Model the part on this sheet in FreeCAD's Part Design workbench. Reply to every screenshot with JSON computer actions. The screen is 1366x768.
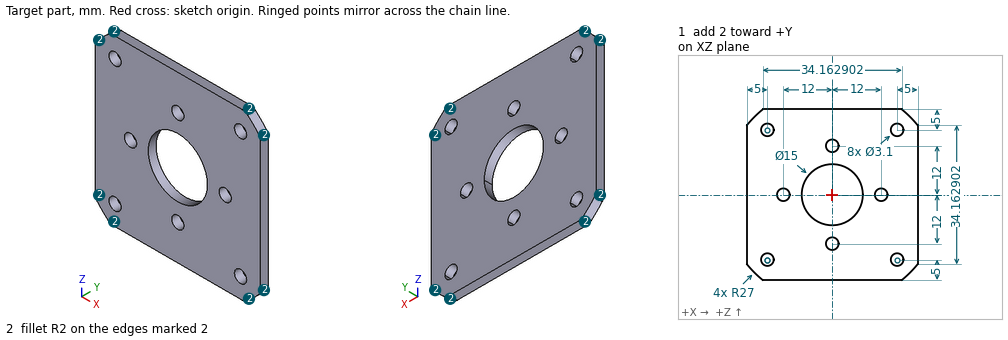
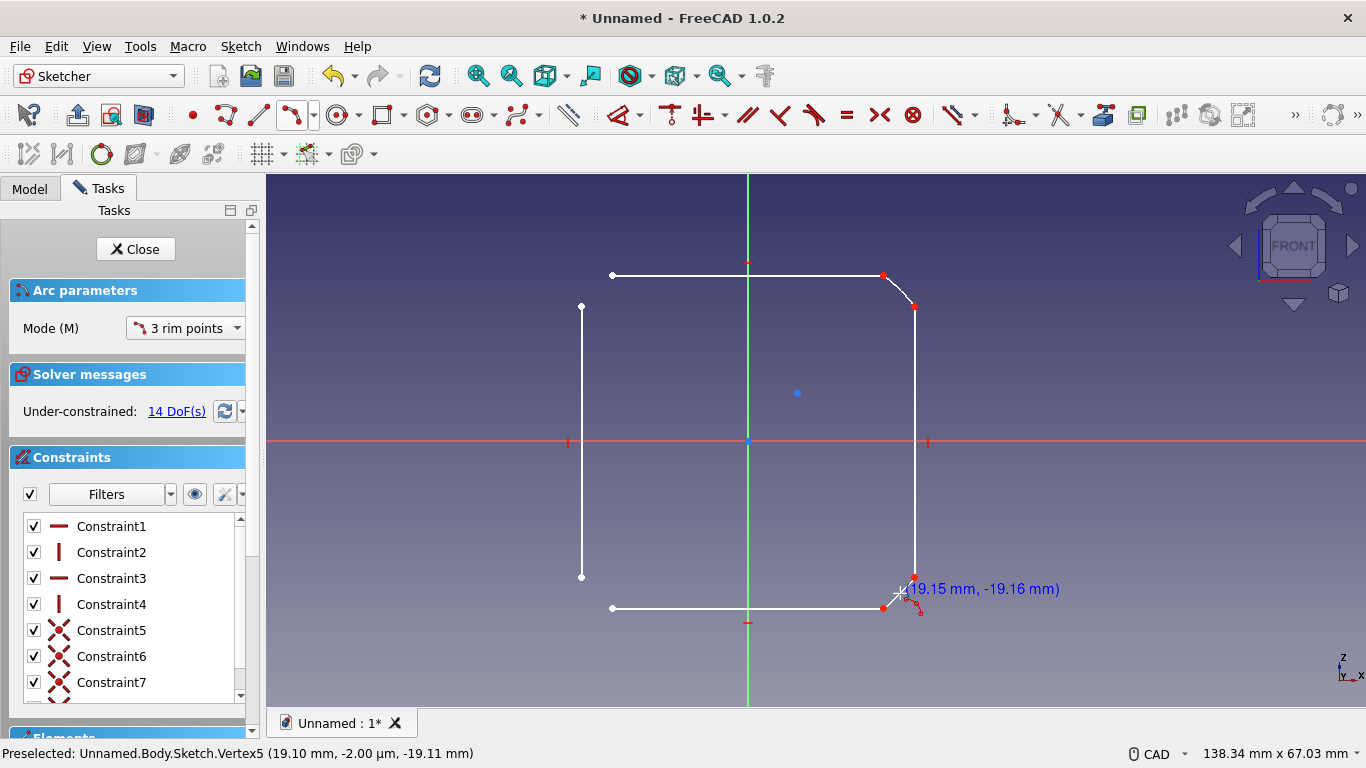
{"action": "left_click", "coordinate": [613, 609]}
{"action": "left_click", "coordinate": [582, 578]}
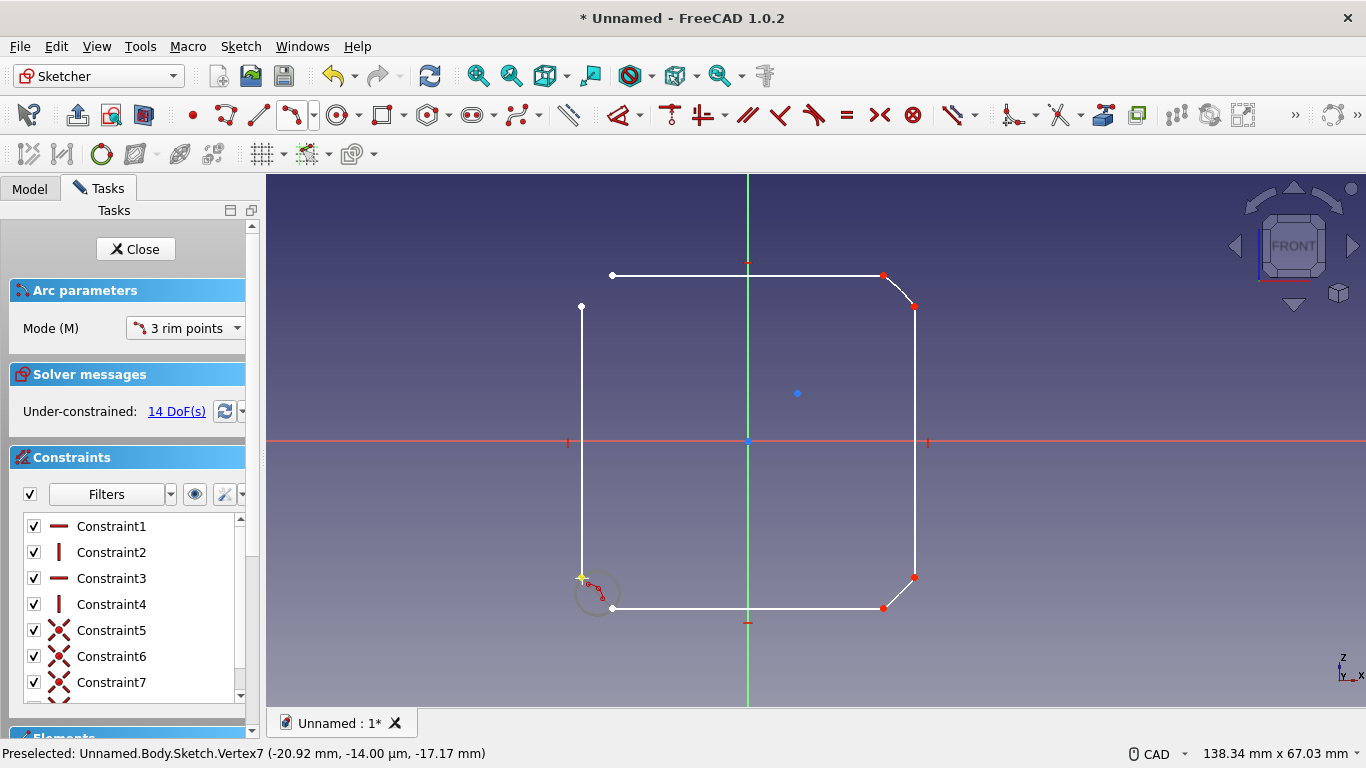
{"action": "scroll", "coordinate": [596, 593], "scroll_direction": "up", "scroll_amount": 14}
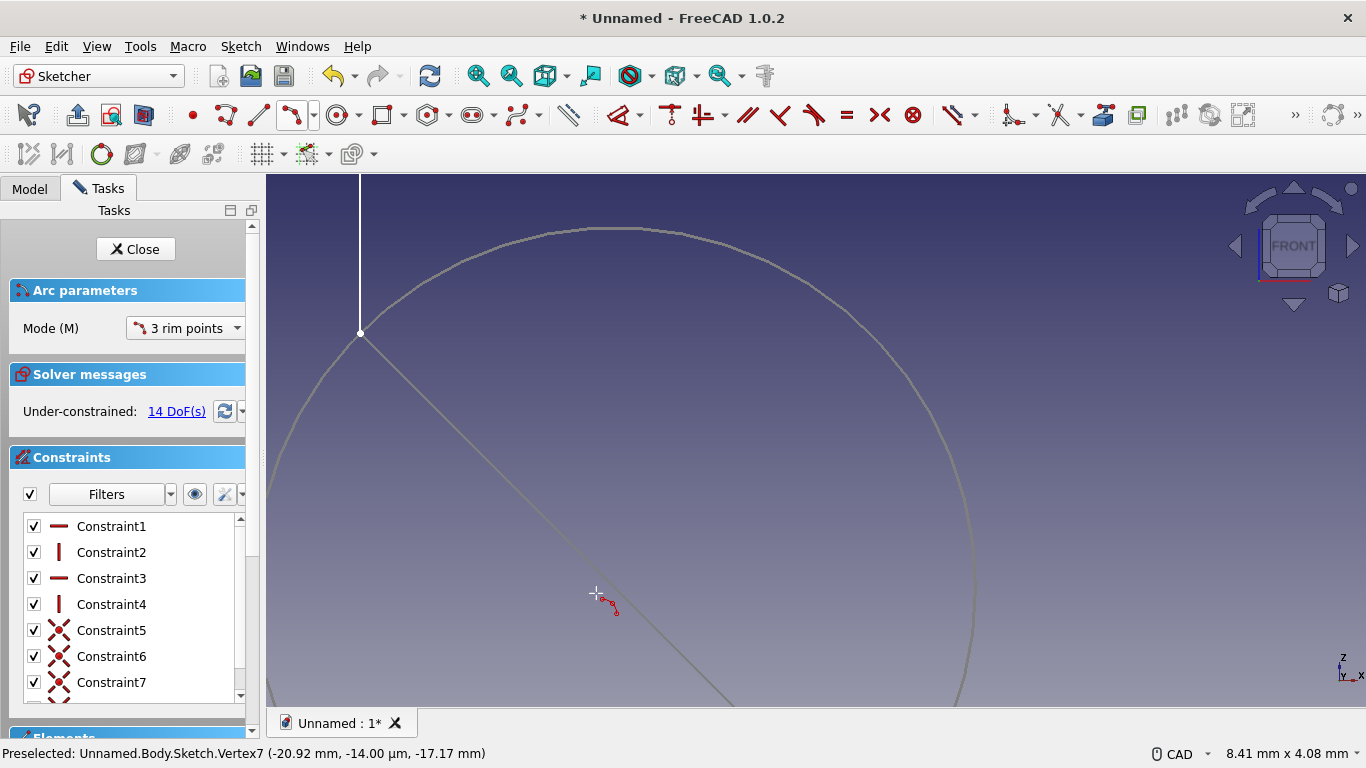
{"action": "left_click", "coordinate": [599, 585]}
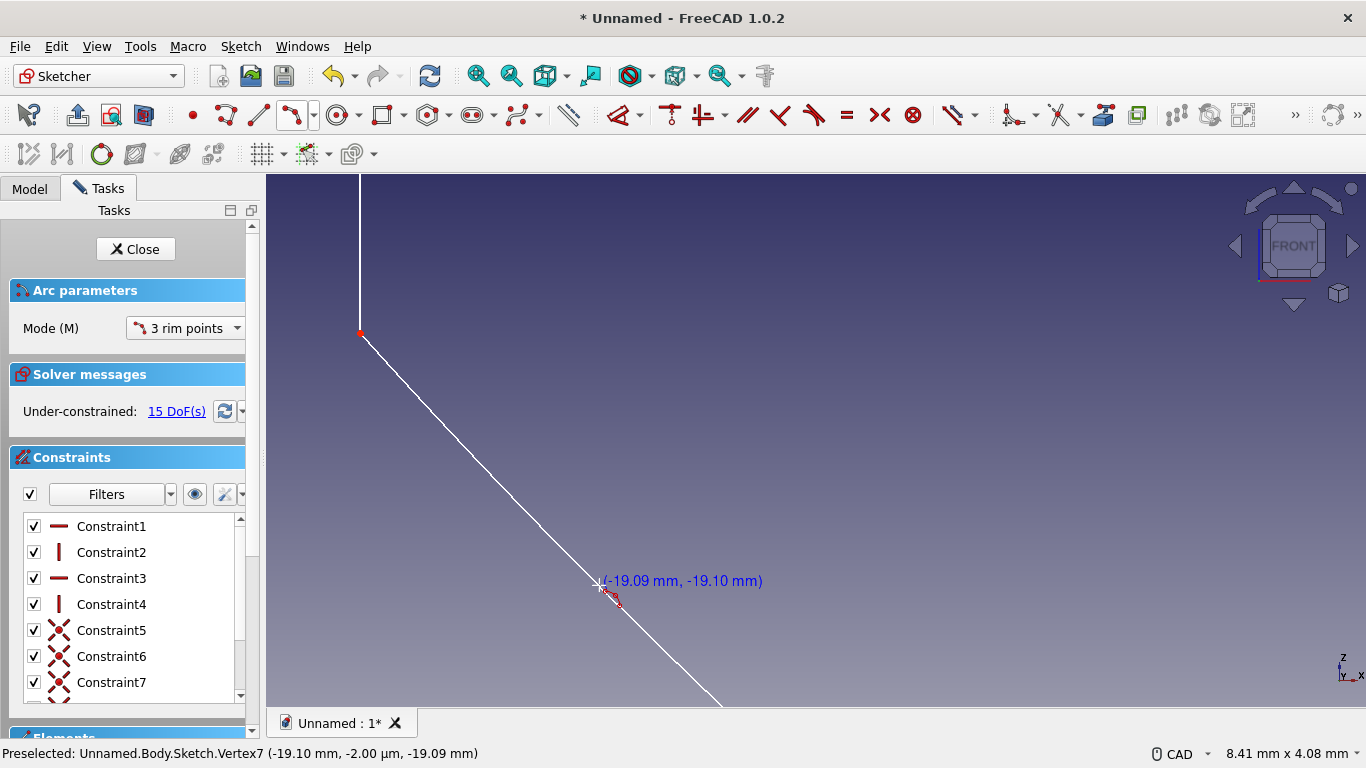
{"action": "scroll", "coordinate": [595, 593], "scroll_direction": "down", "scroll_amount": 14}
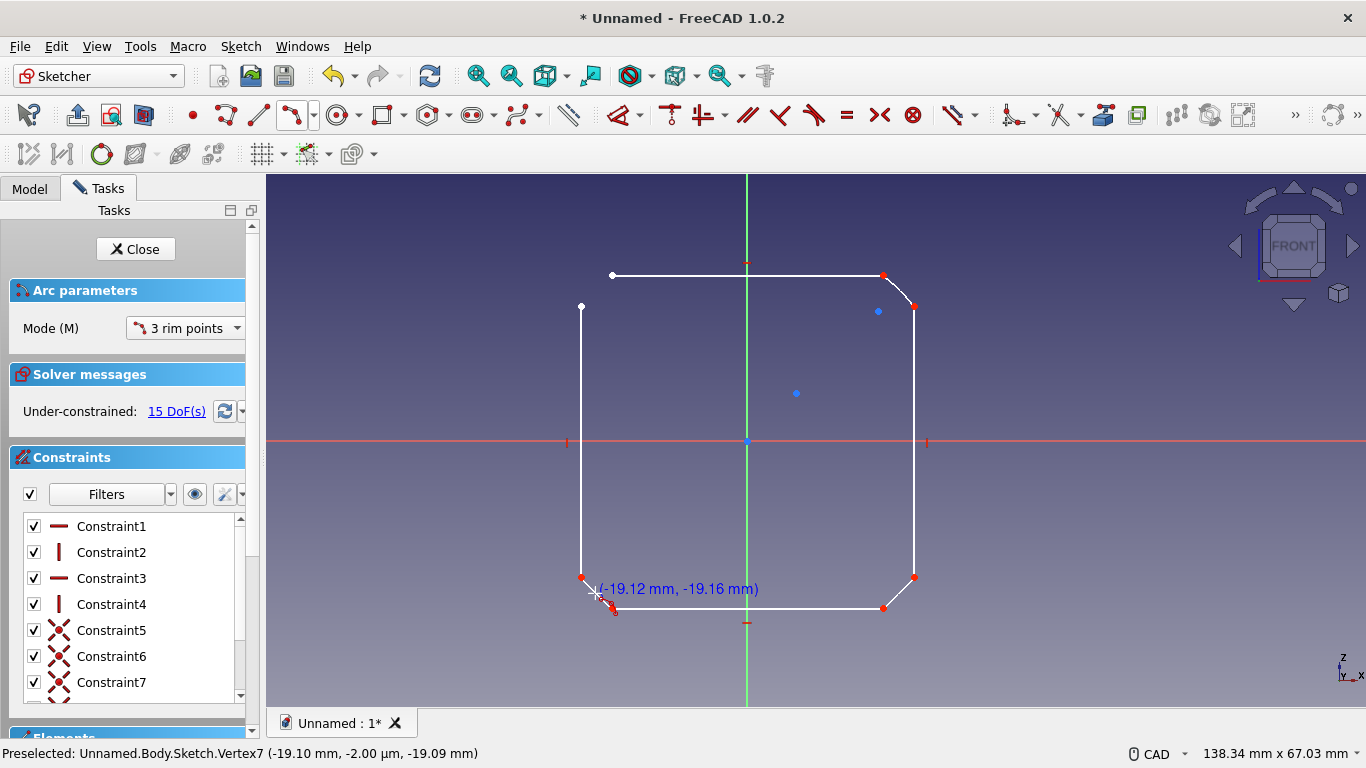
{"action": "left_click", "coordinate": [581, 307]}
{"action": "left_click", "coordinate": [612, 276]}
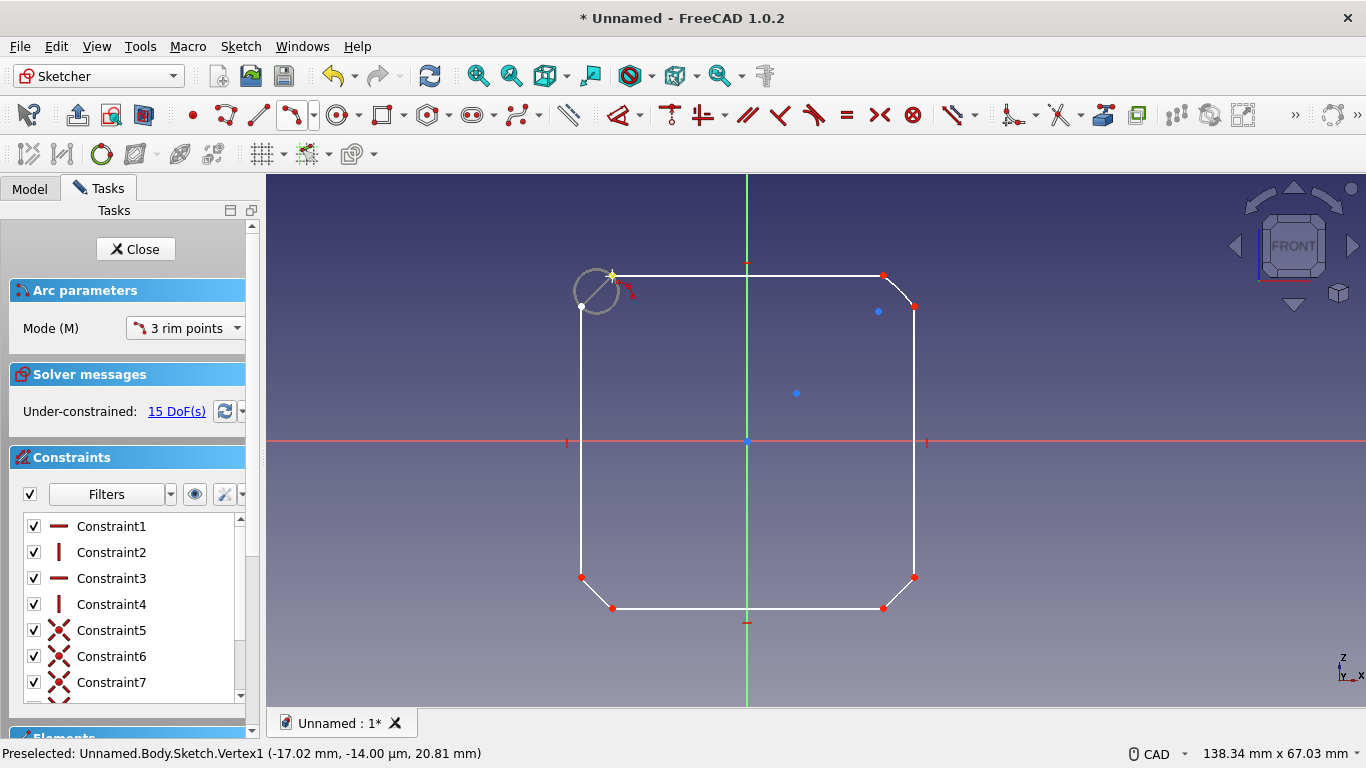
{"action": "scroll", "coordinate": [596, 290], "scroll_direction": "up", "scroll_amount": 14}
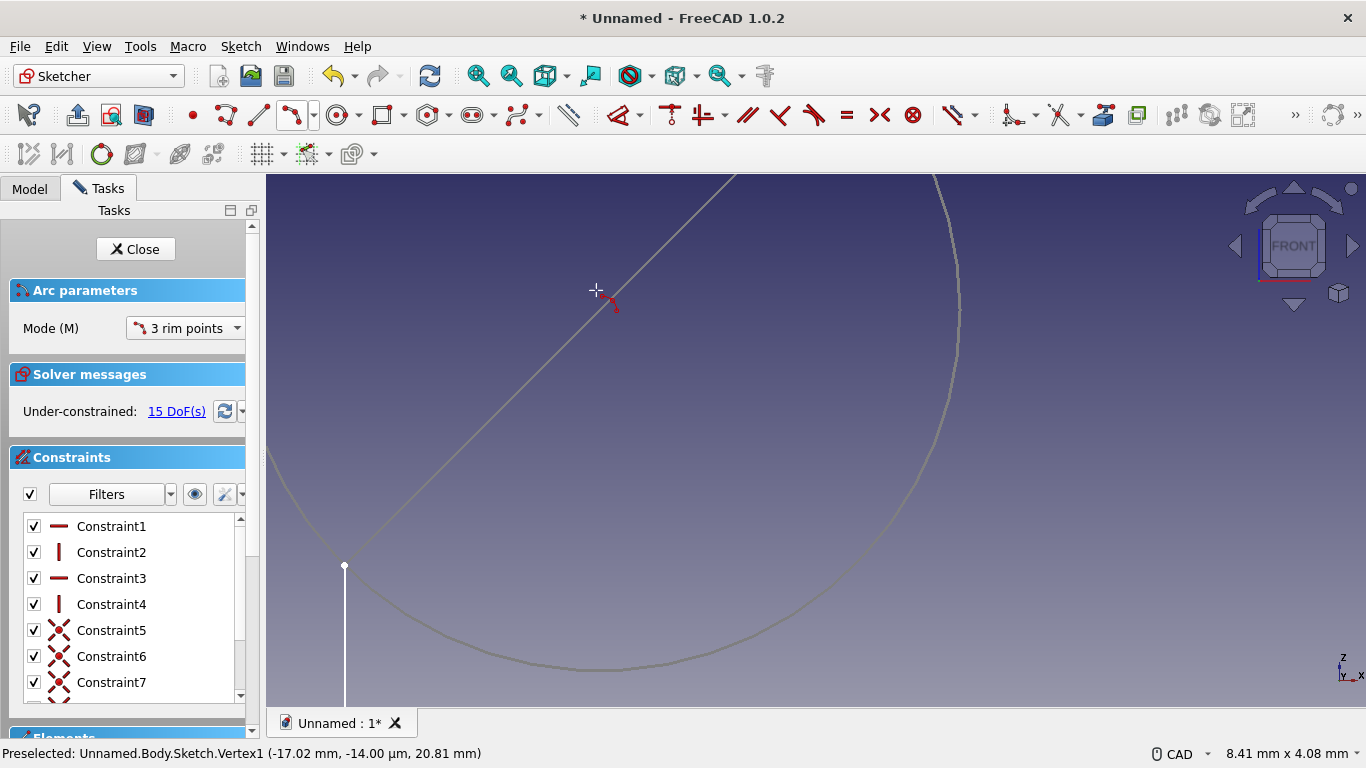
{"action": "left_click", "coordinate": [583, 281]}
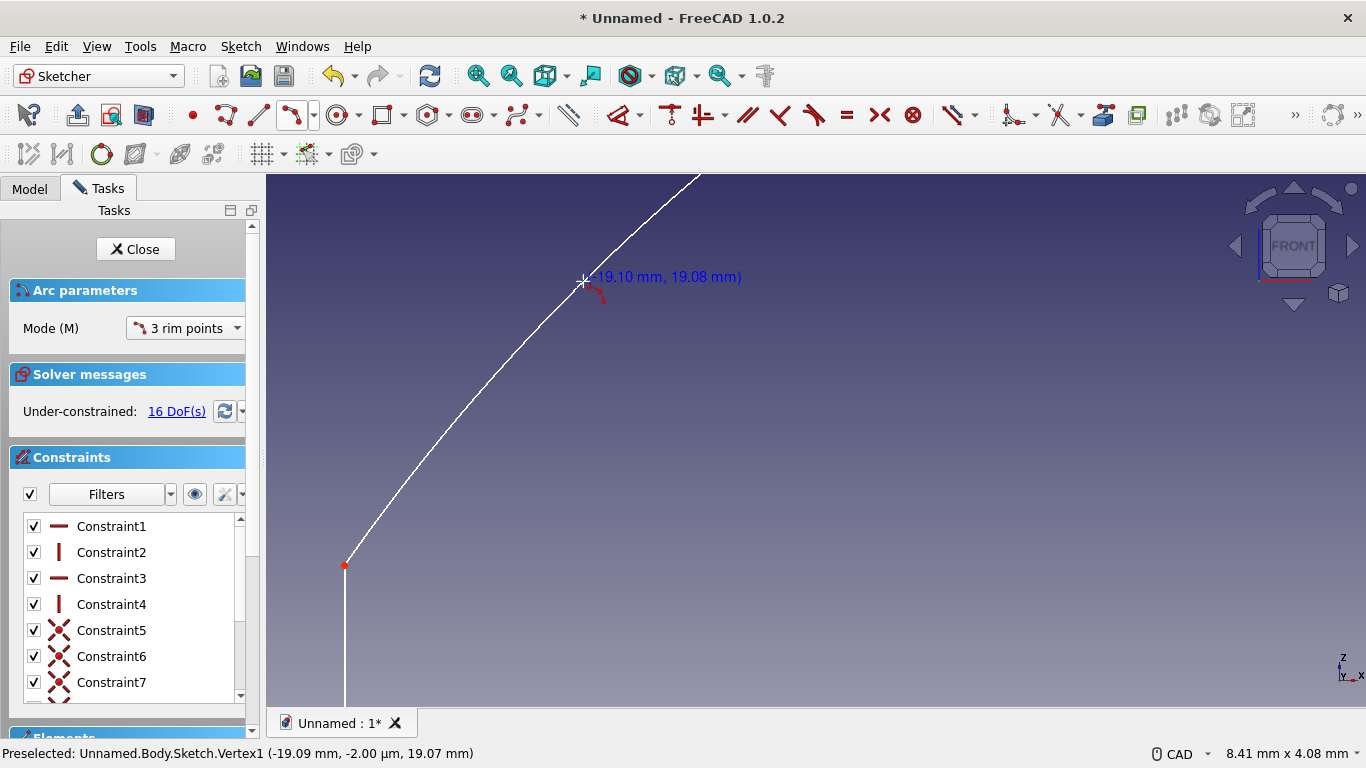
{"action": "left_click", "coordinate": [336, 116]}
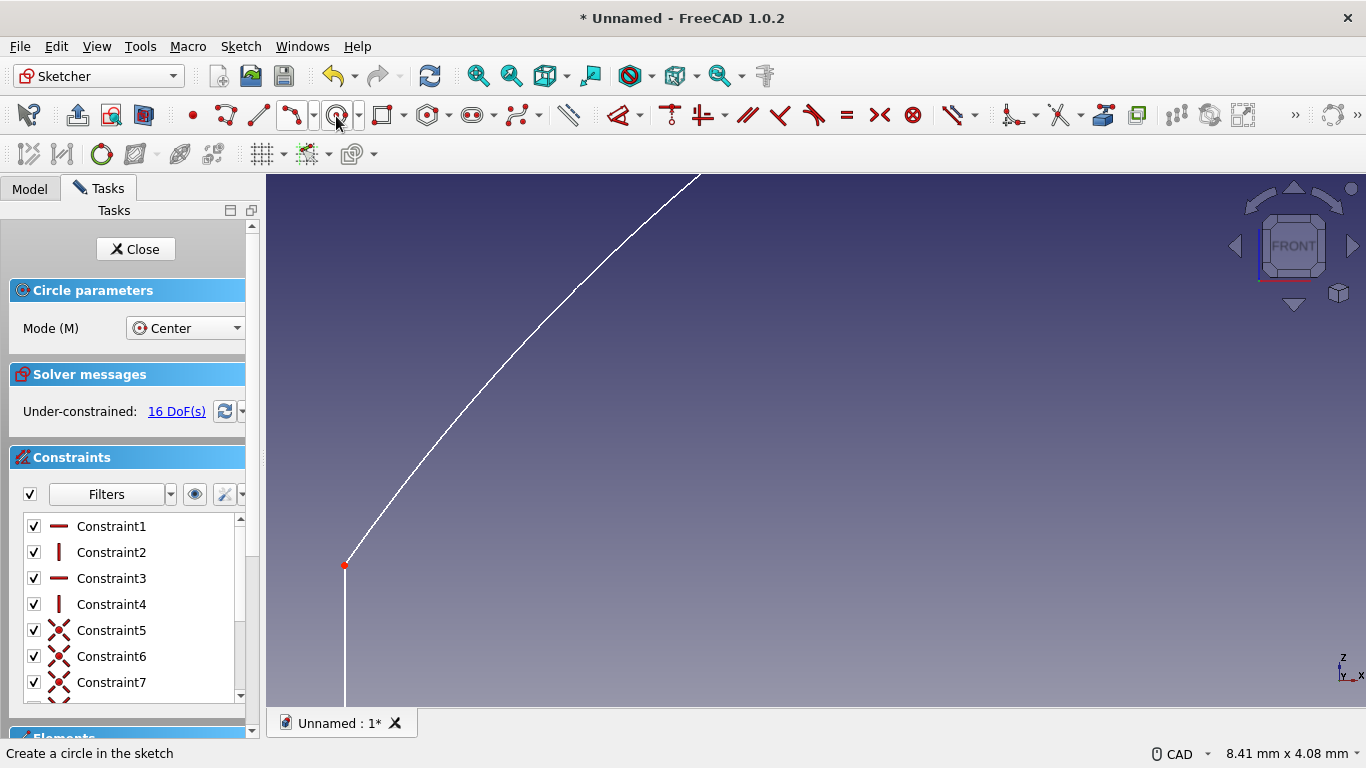
{"action": "scroll", "coordinate": [596, 289], "scroll_direction": "down", "scroll_amount": 14}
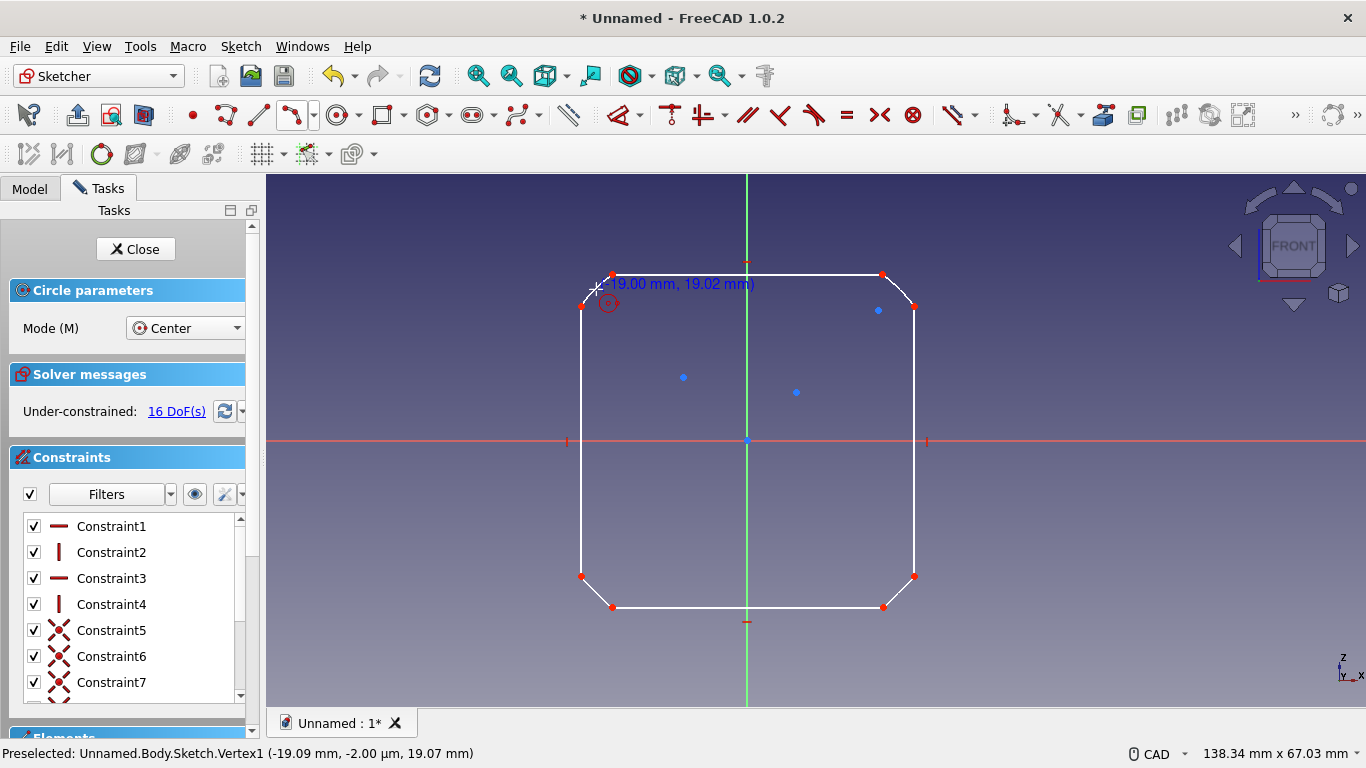
{"action": "scroll", "coordinate": [874, 314], "scroll_direction": "up", "scroll_amount": 4}